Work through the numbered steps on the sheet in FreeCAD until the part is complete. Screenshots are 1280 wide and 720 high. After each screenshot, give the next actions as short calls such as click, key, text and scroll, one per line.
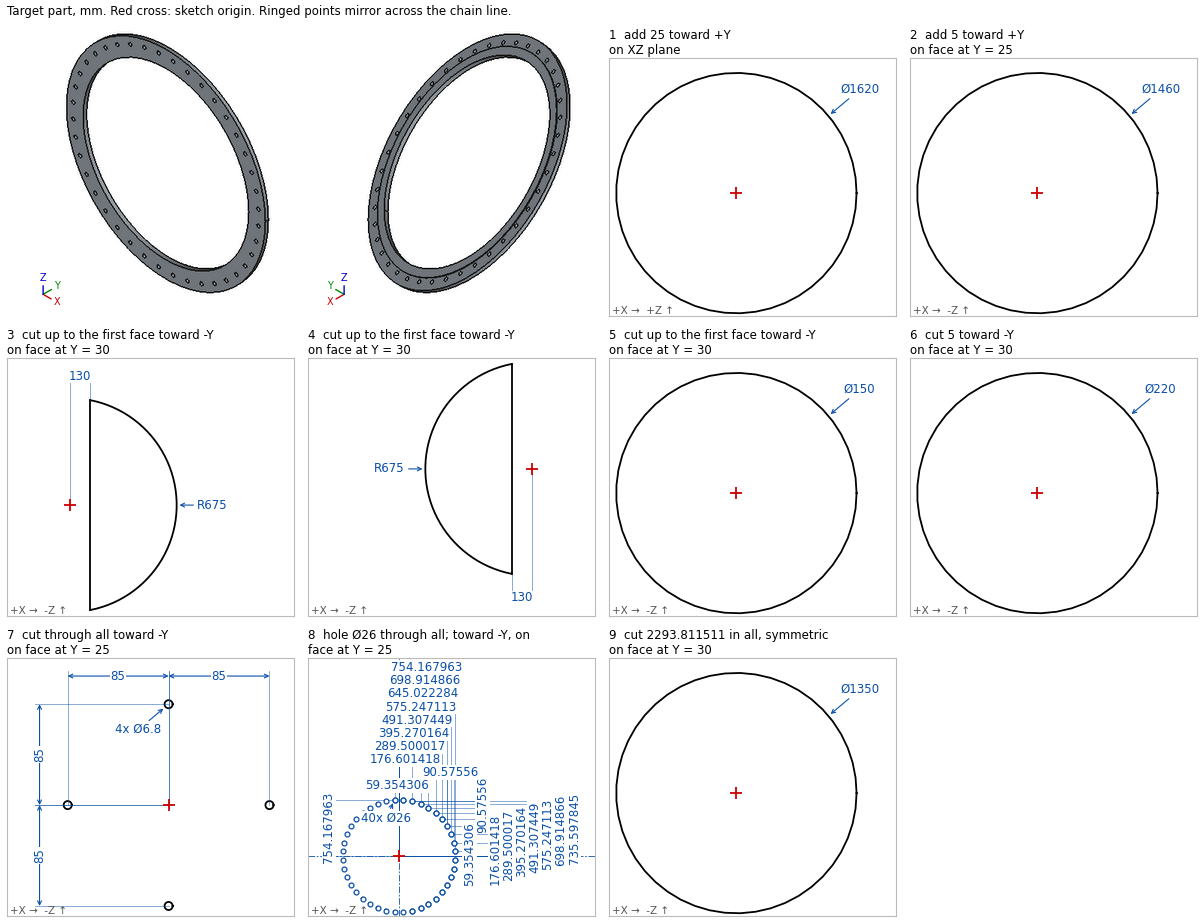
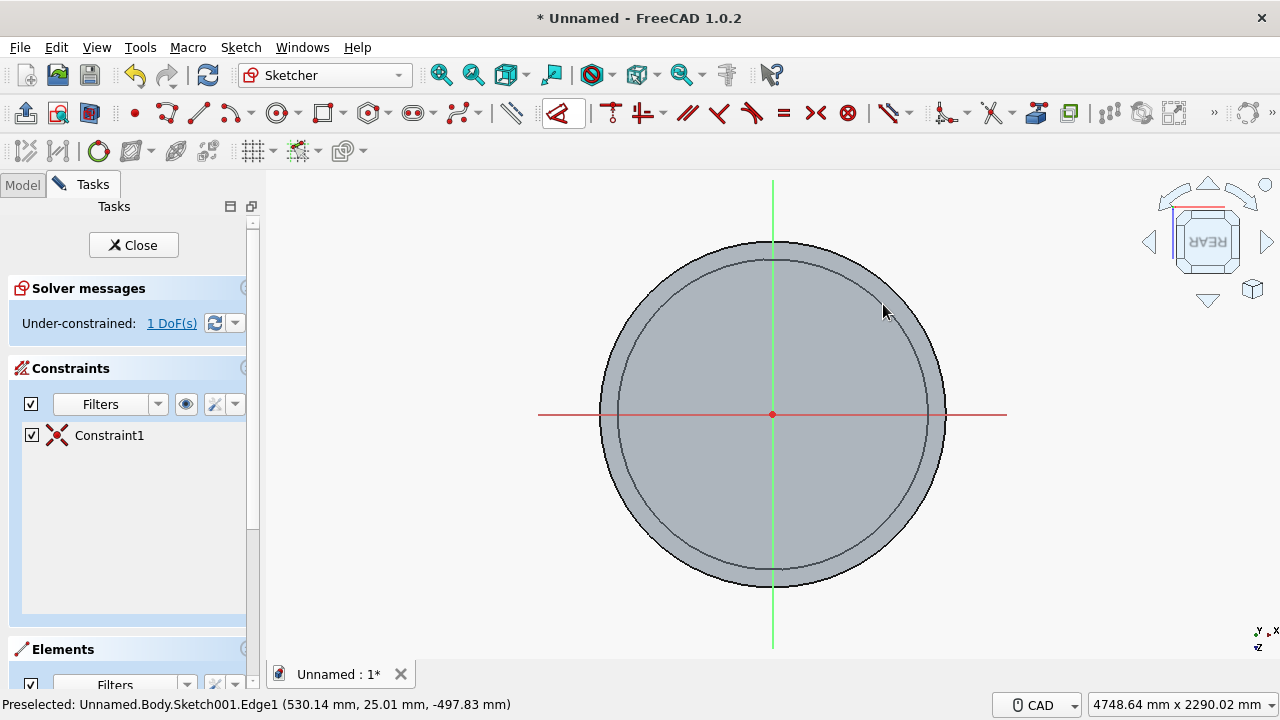
click(882, 304)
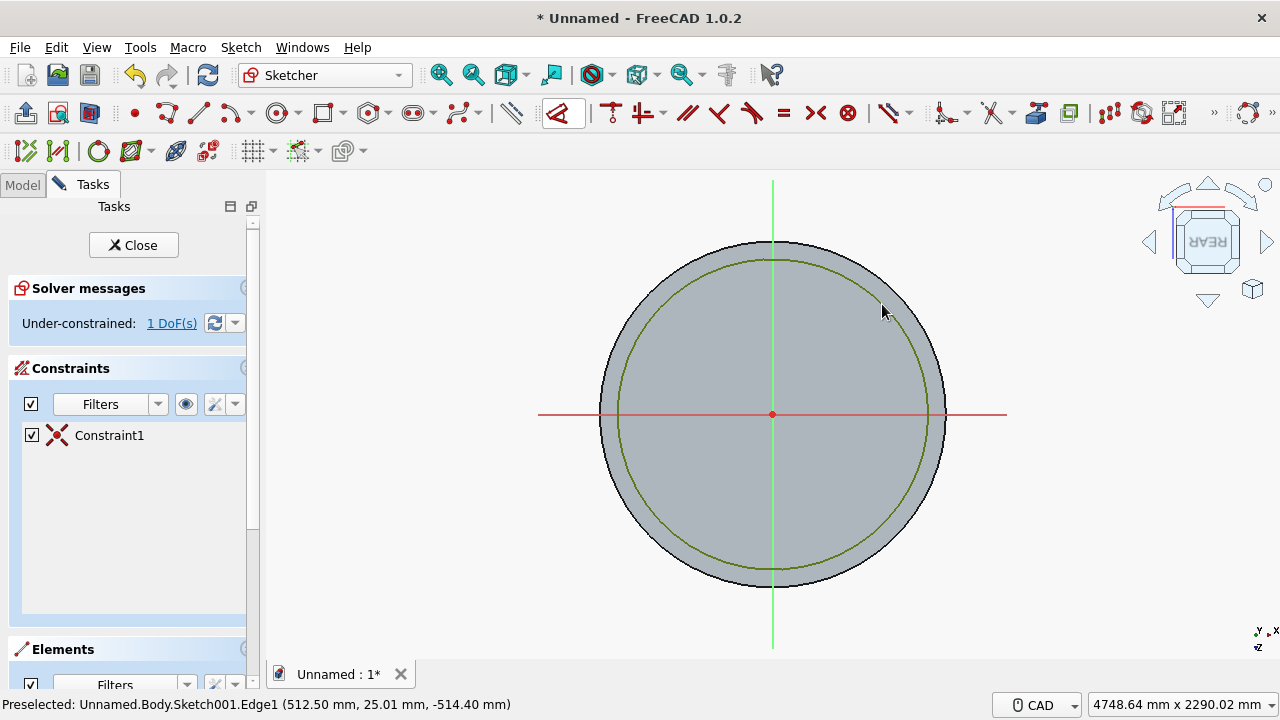
click(580, 114)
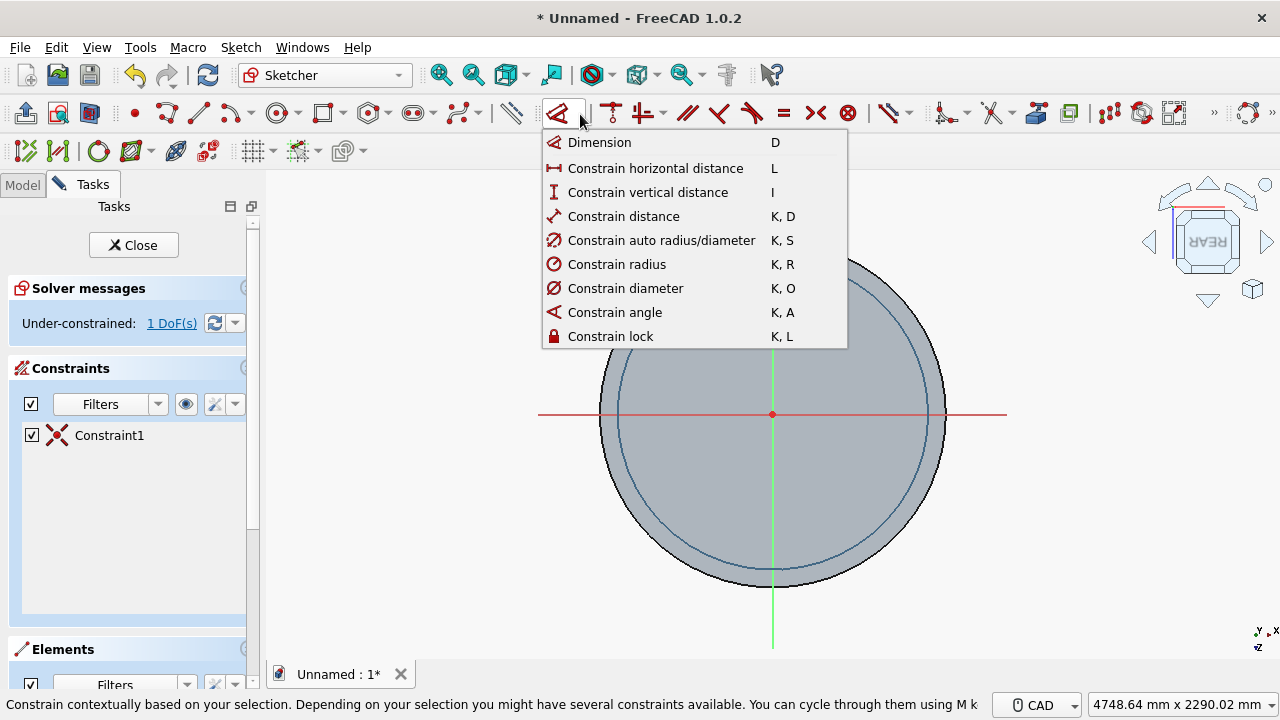
click(695, 288)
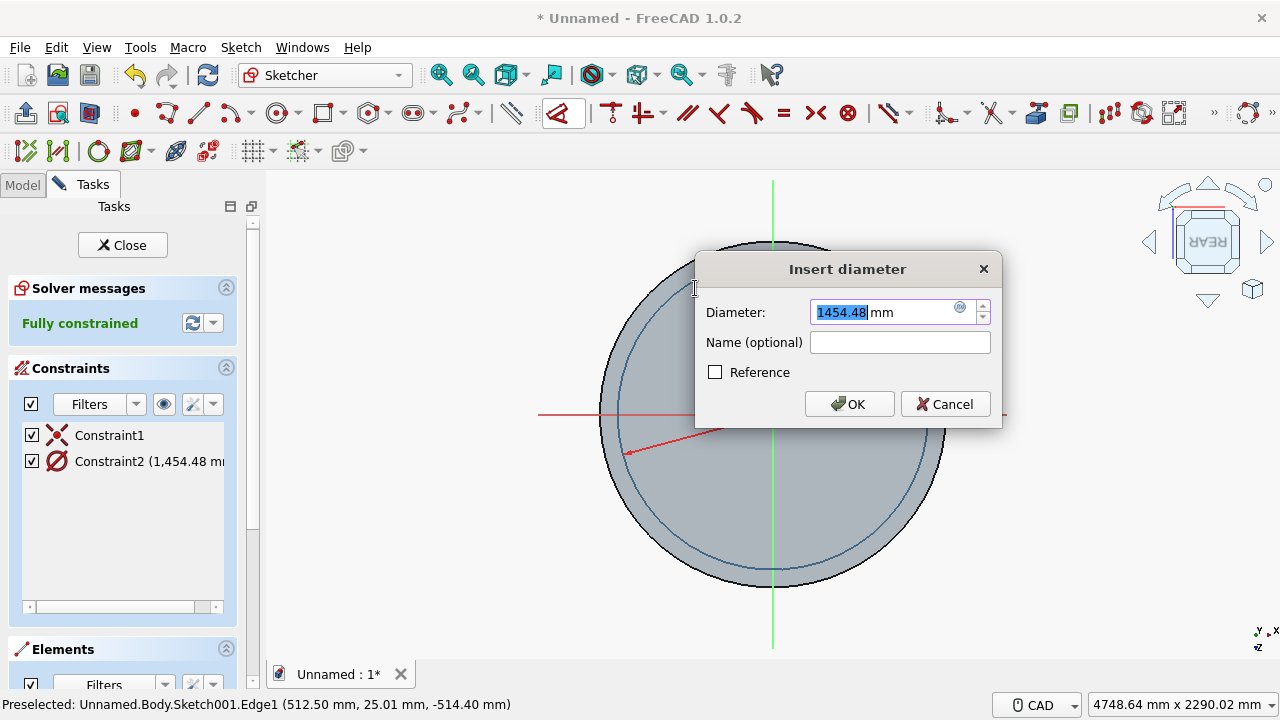
text(1460)
key(Return)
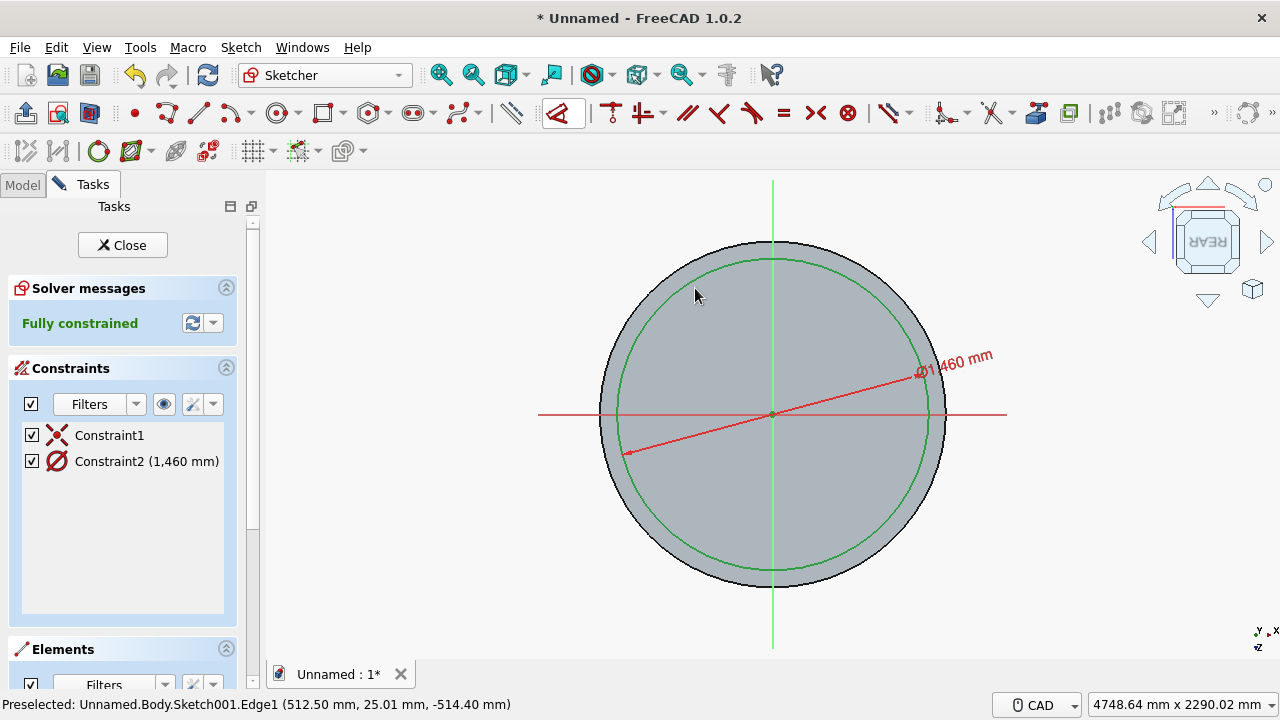
click(123, 245)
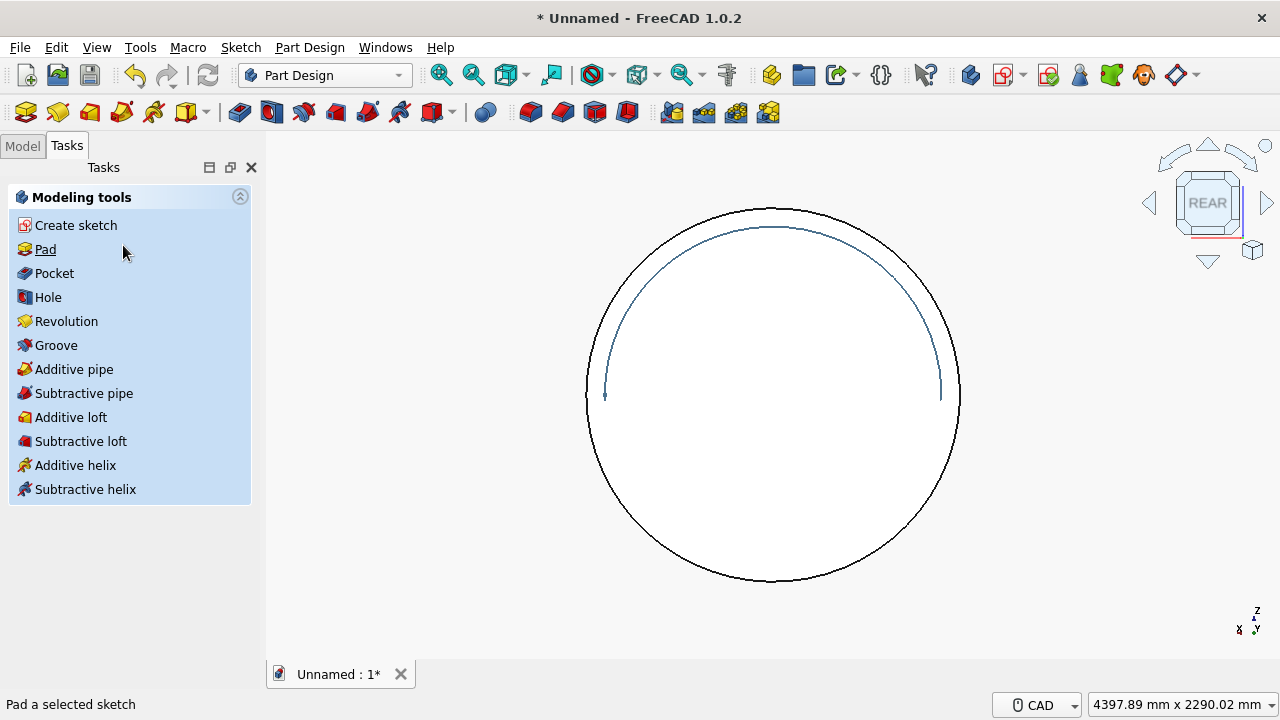
click(26, 112)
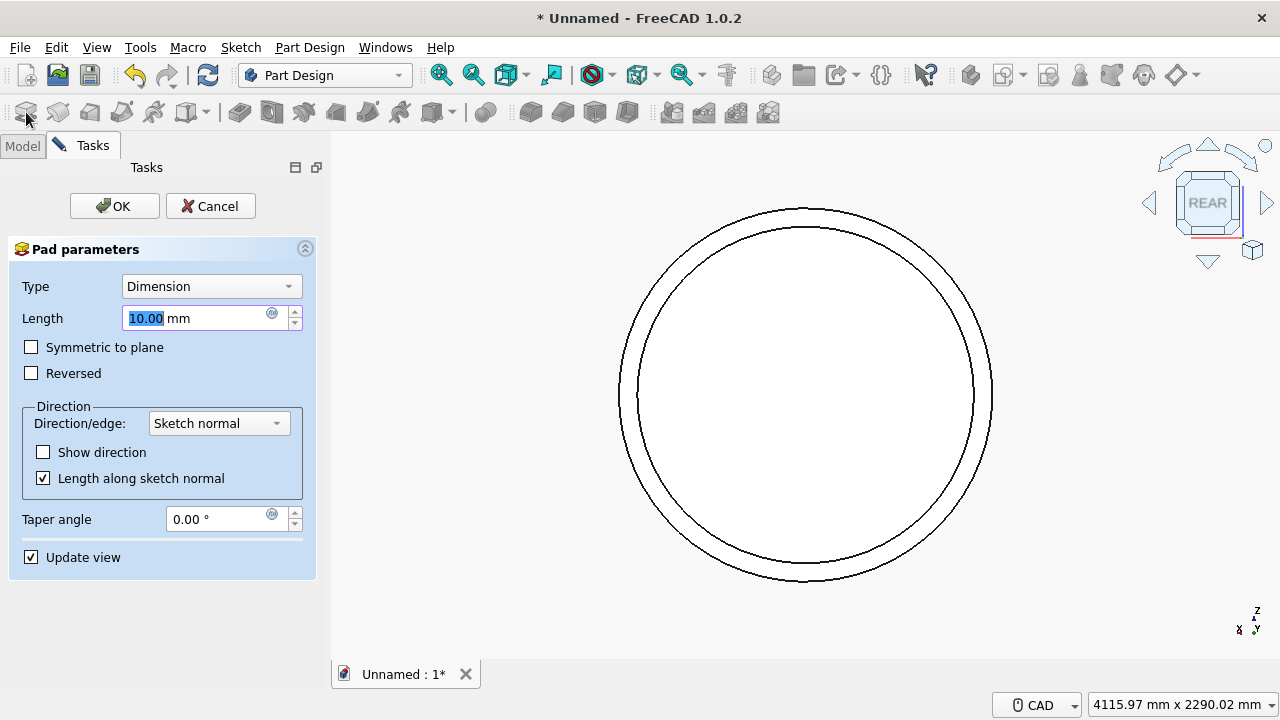
text(5)
key(Tab)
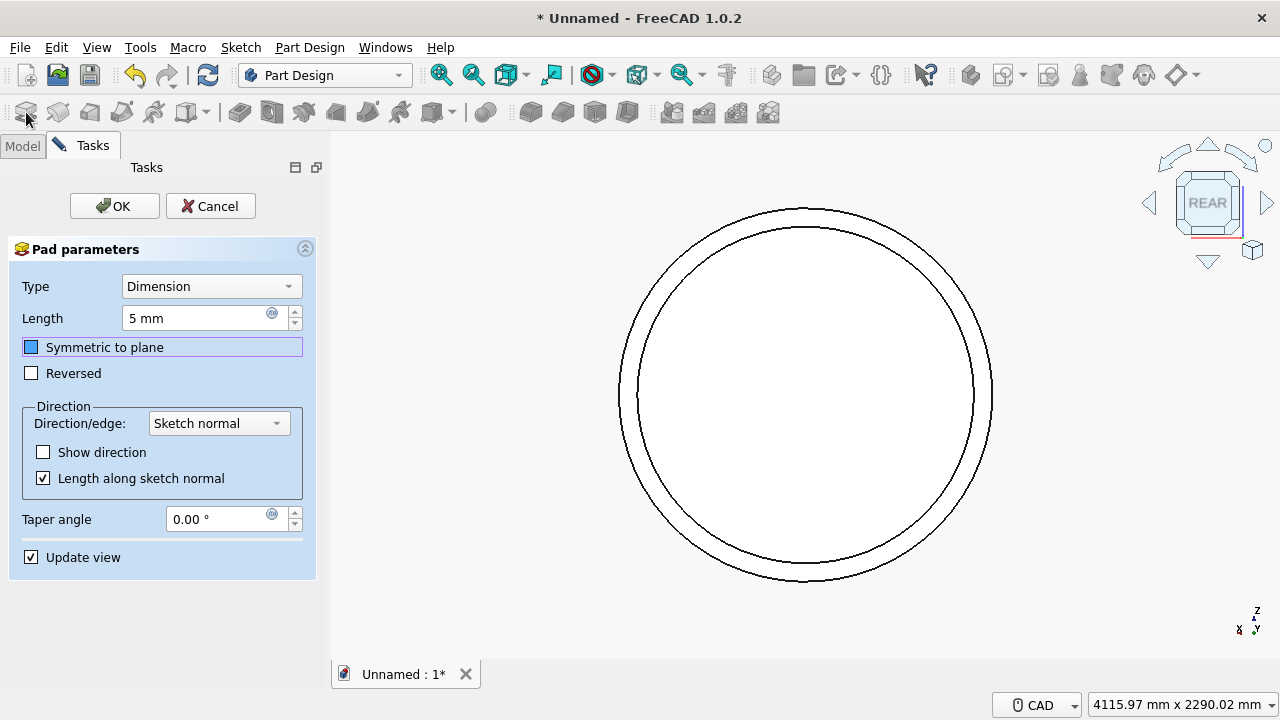
click(115, 206)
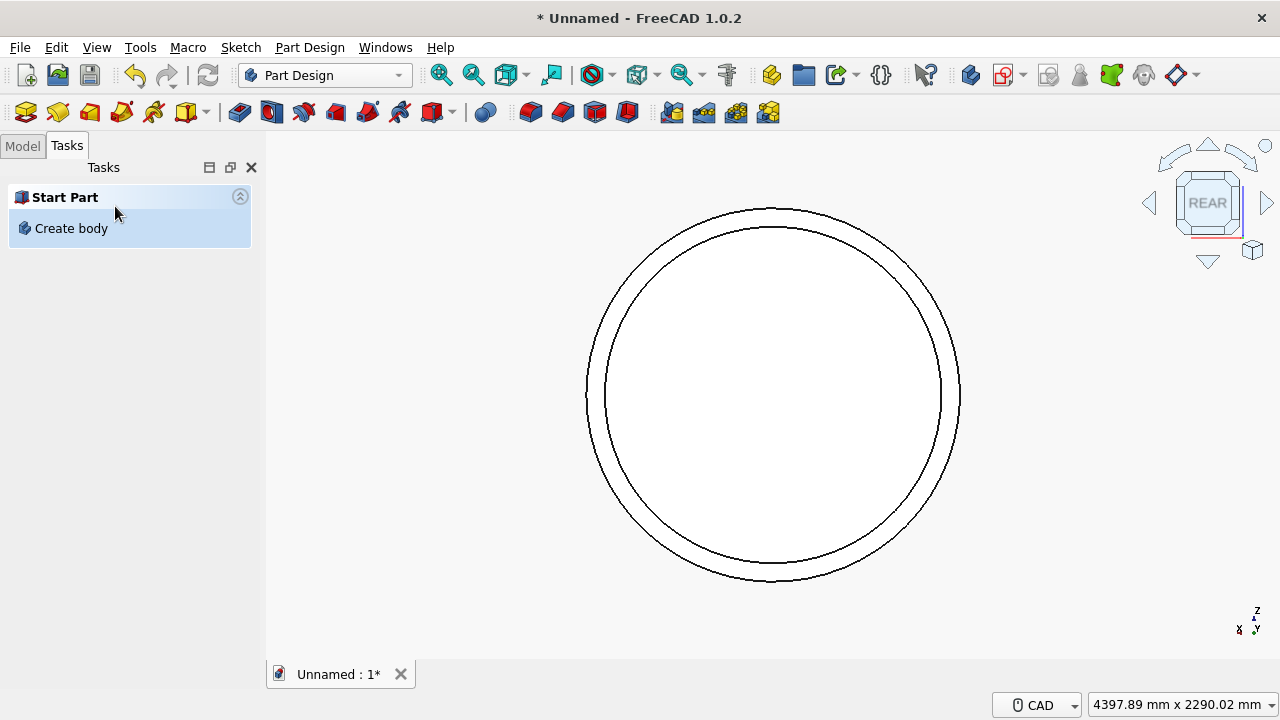
click(773, 394)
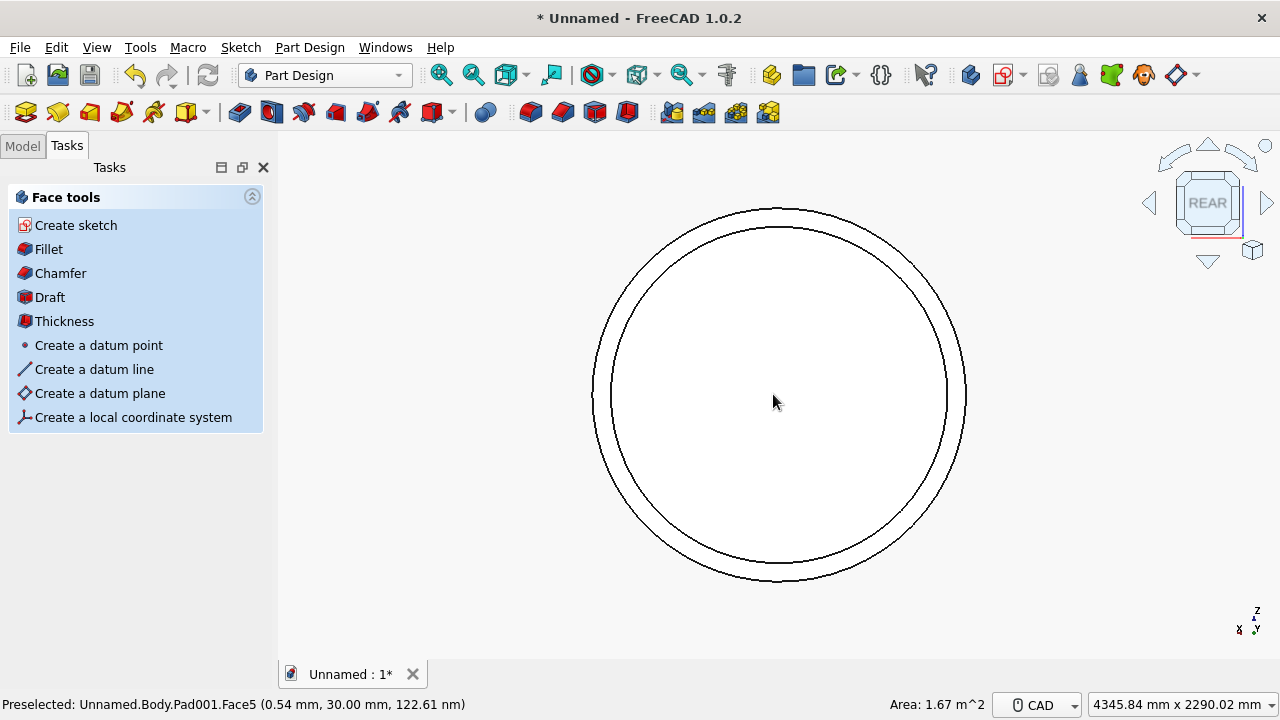
click(1004, 76)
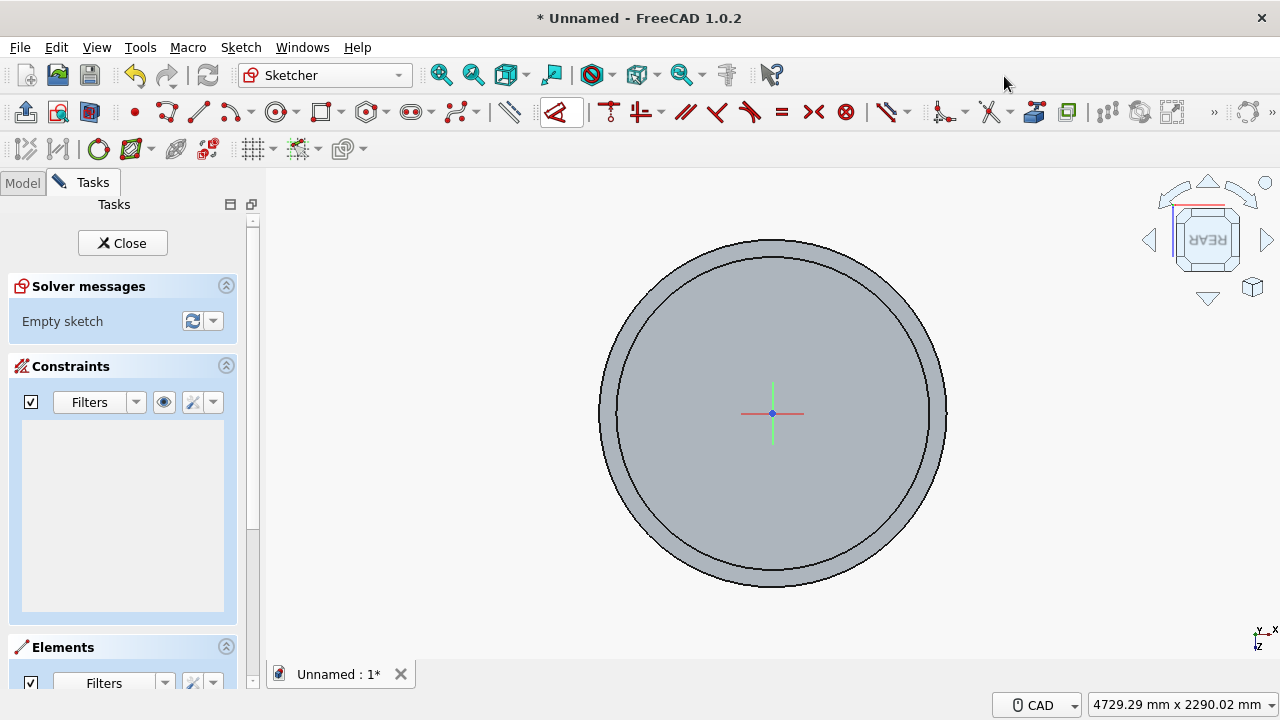
key(g)
key(l)